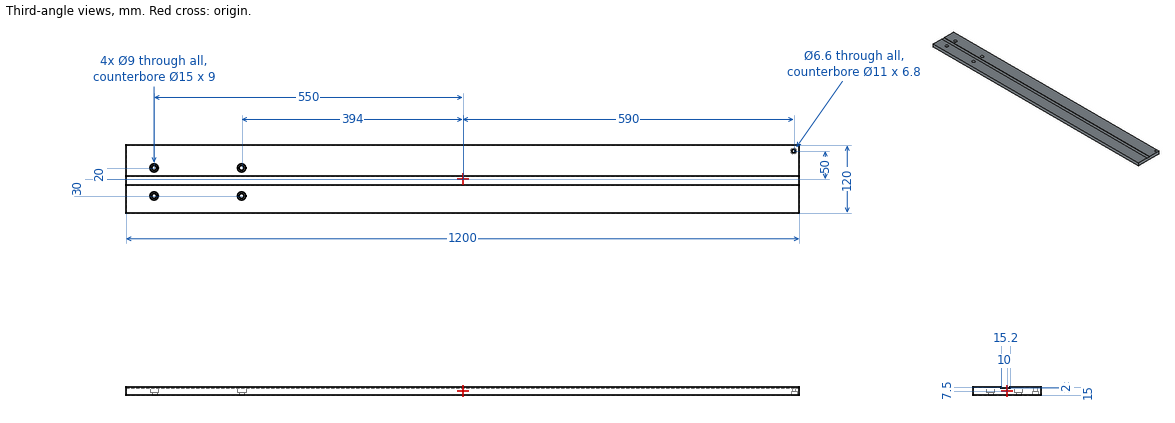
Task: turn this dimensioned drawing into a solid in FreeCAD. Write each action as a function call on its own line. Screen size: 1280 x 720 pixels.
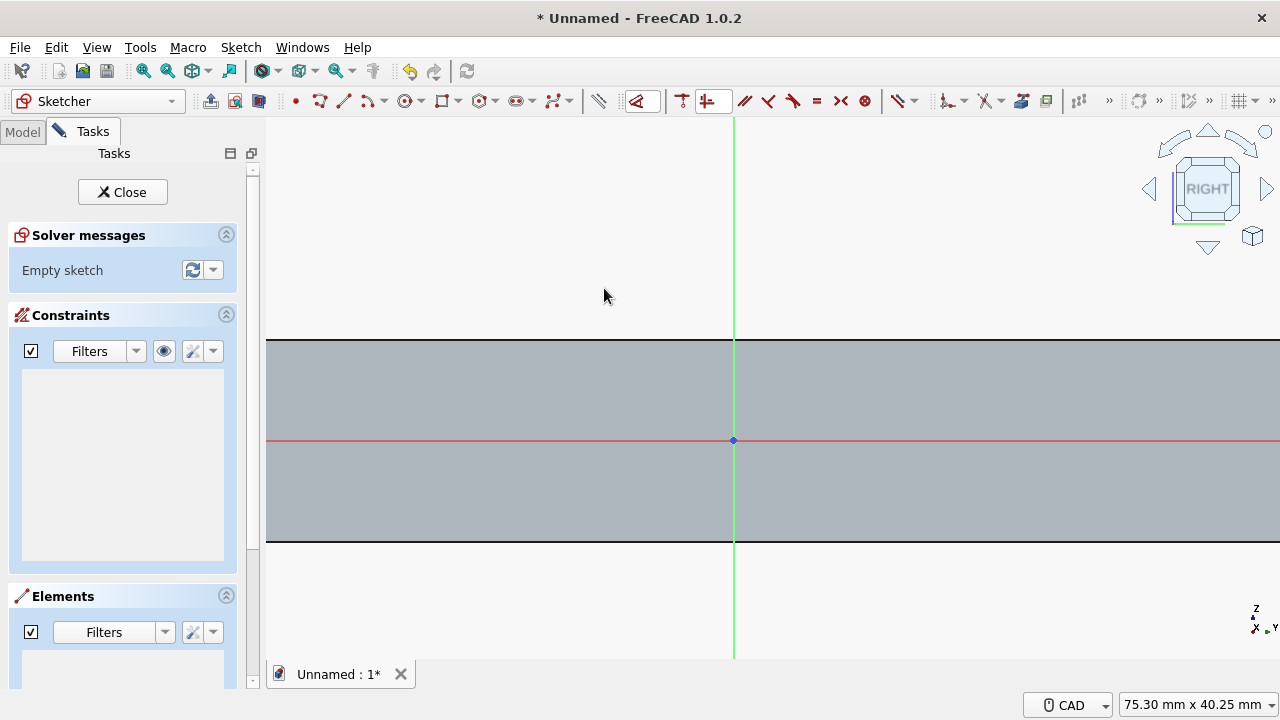
scroll(700, 392, up, 5)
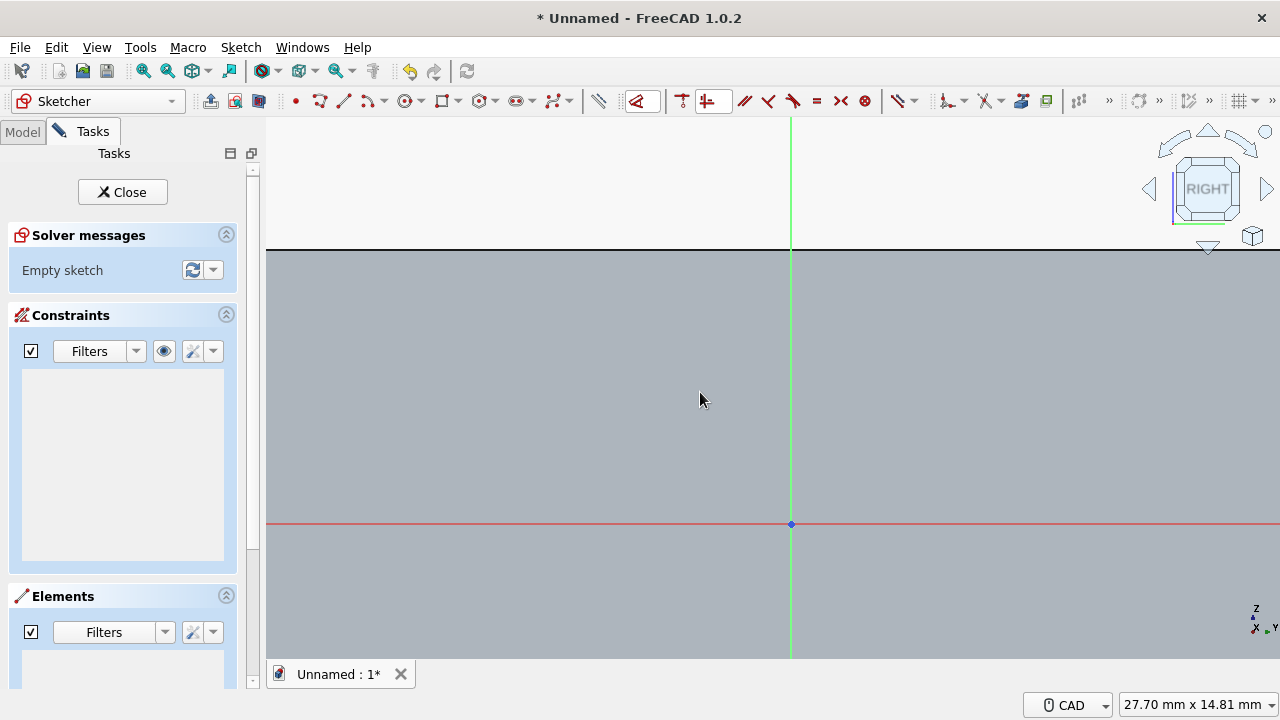
click(442, 102)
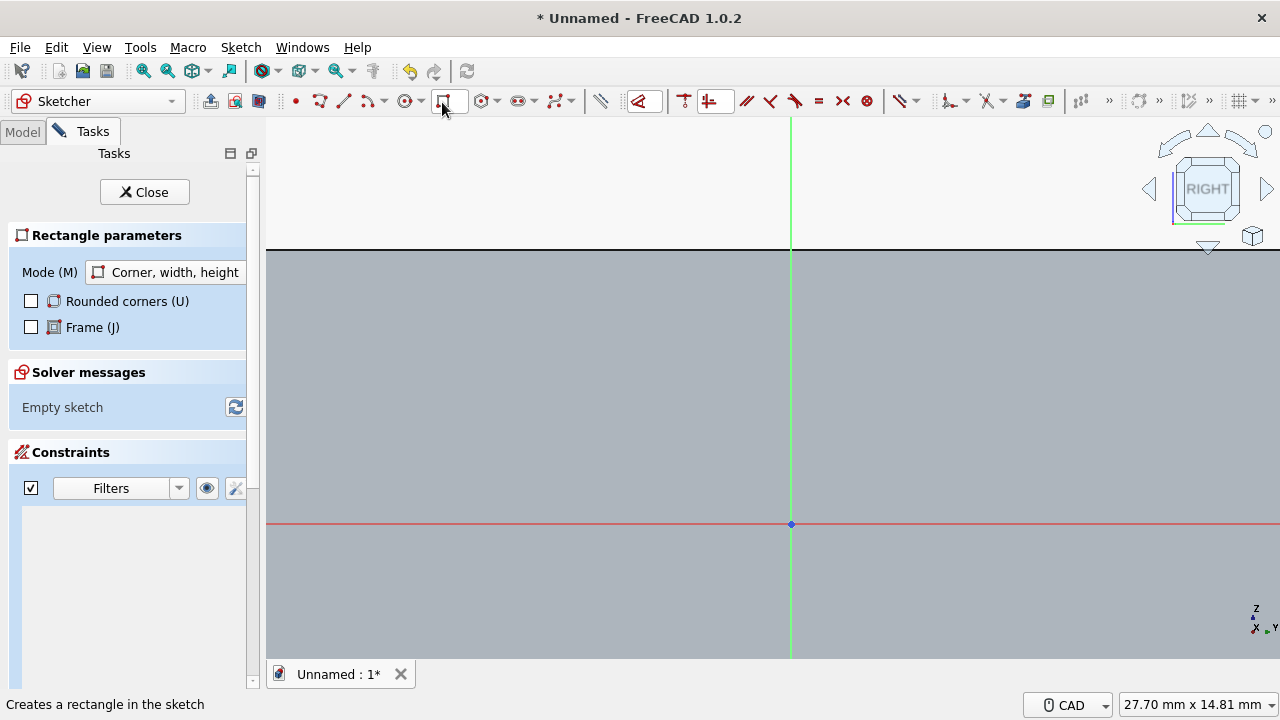
click(425, 250)
move(982, 323)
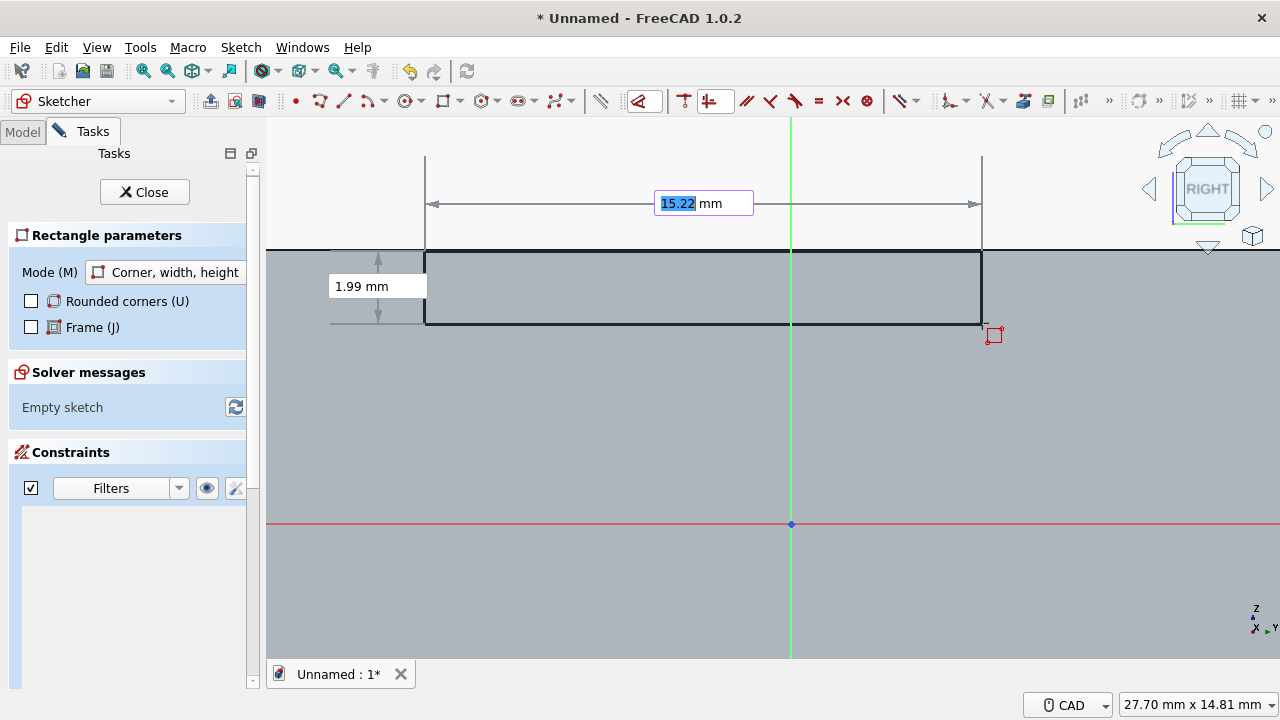
text(15.2)
key(Tab)
text(2)
key(Return)
key(Escape)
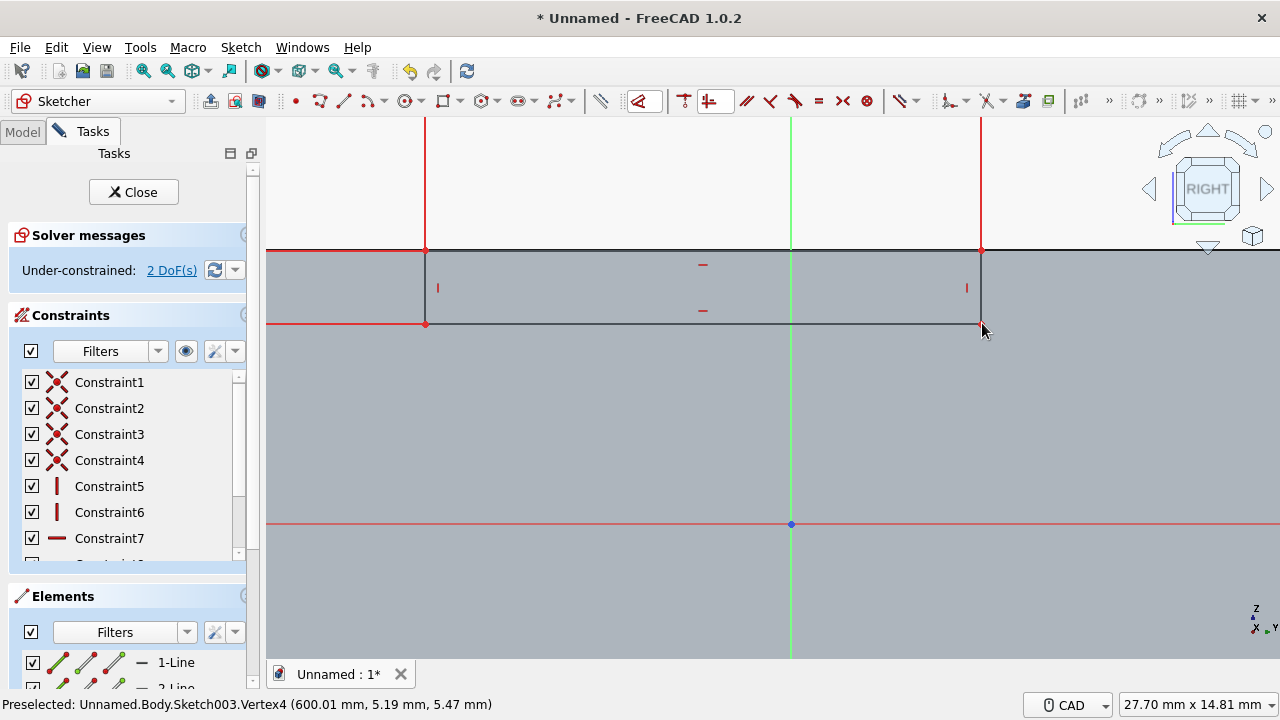
click(425, 251)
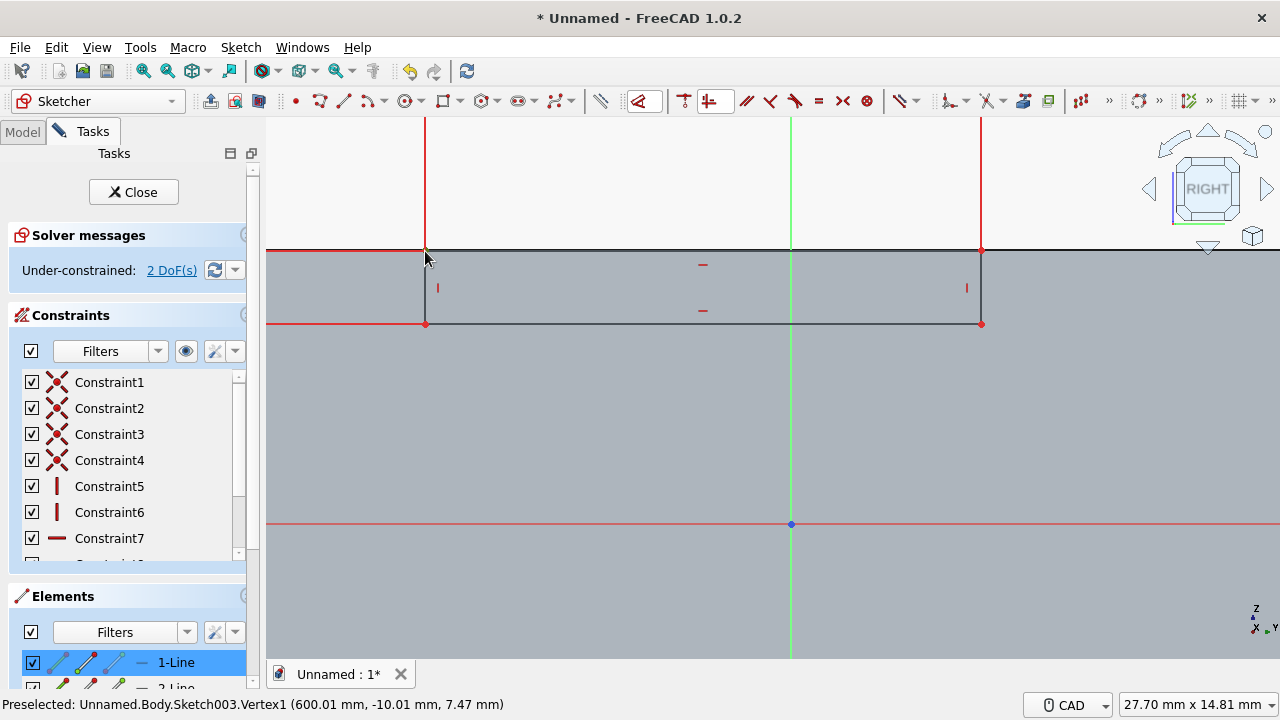
click(656, 102)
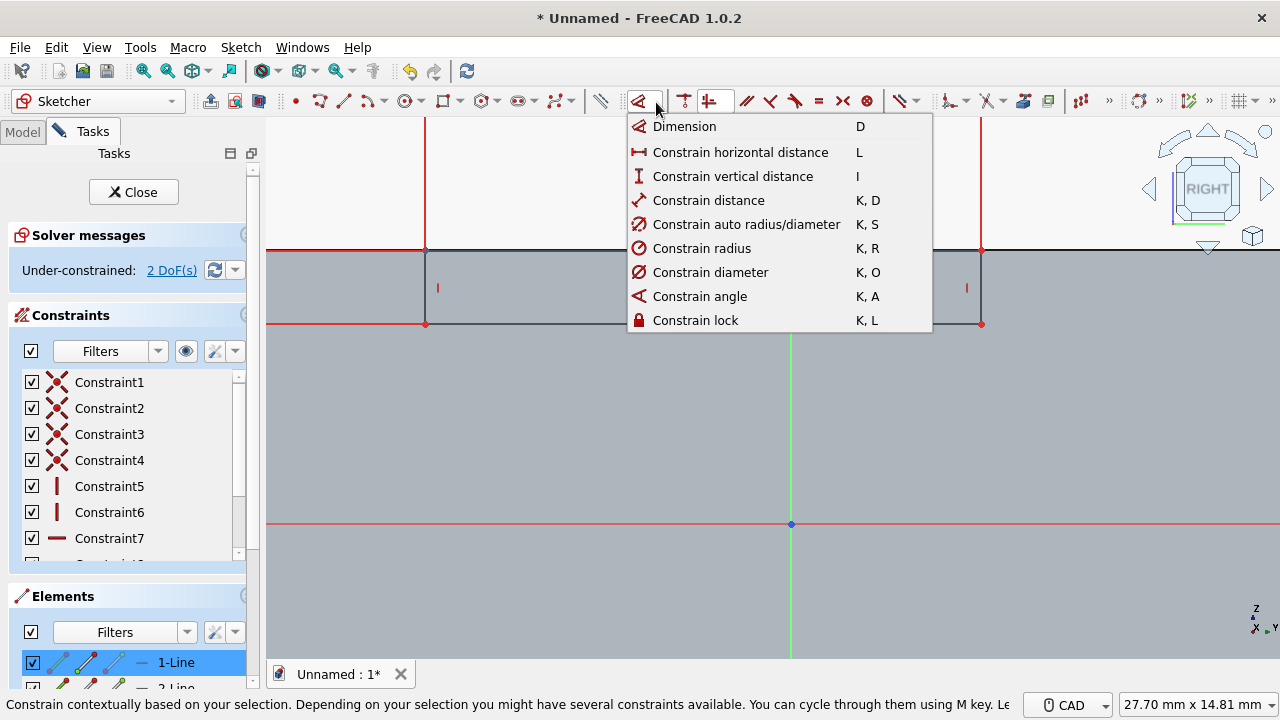
click(780, 152)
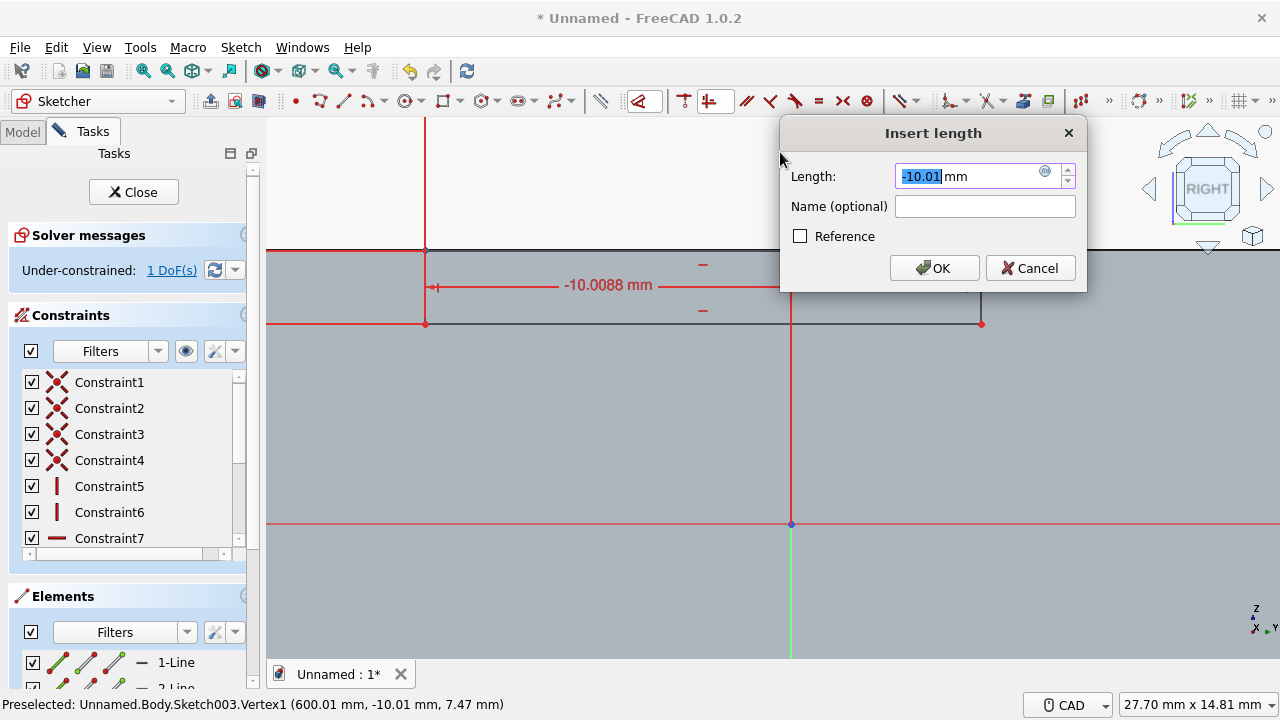
text(-10)
key(Return)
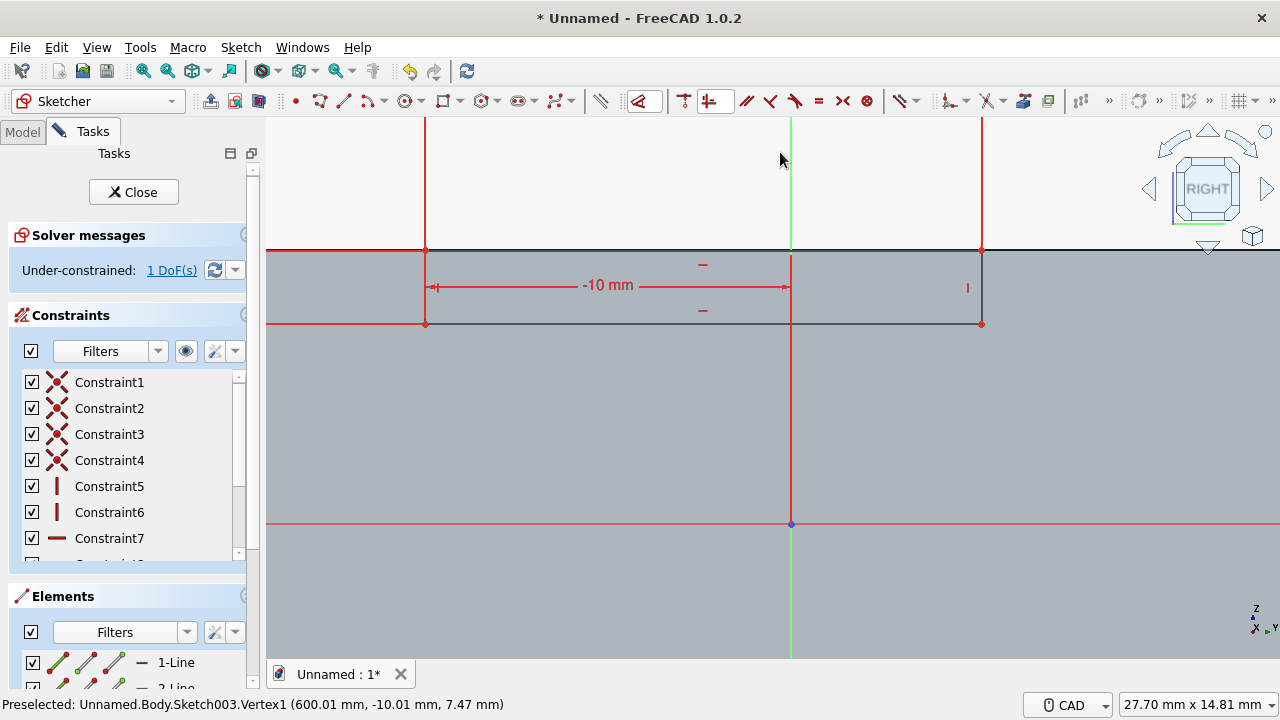
click(425, 251)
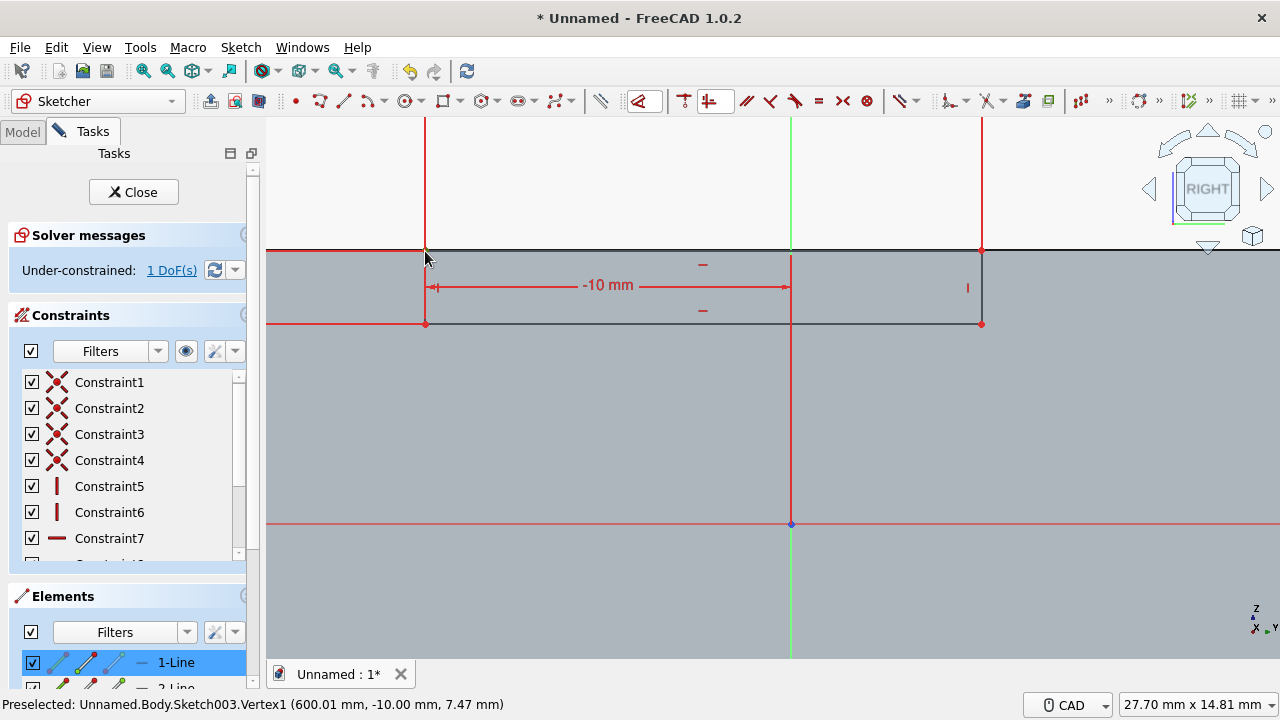
click(656, 102)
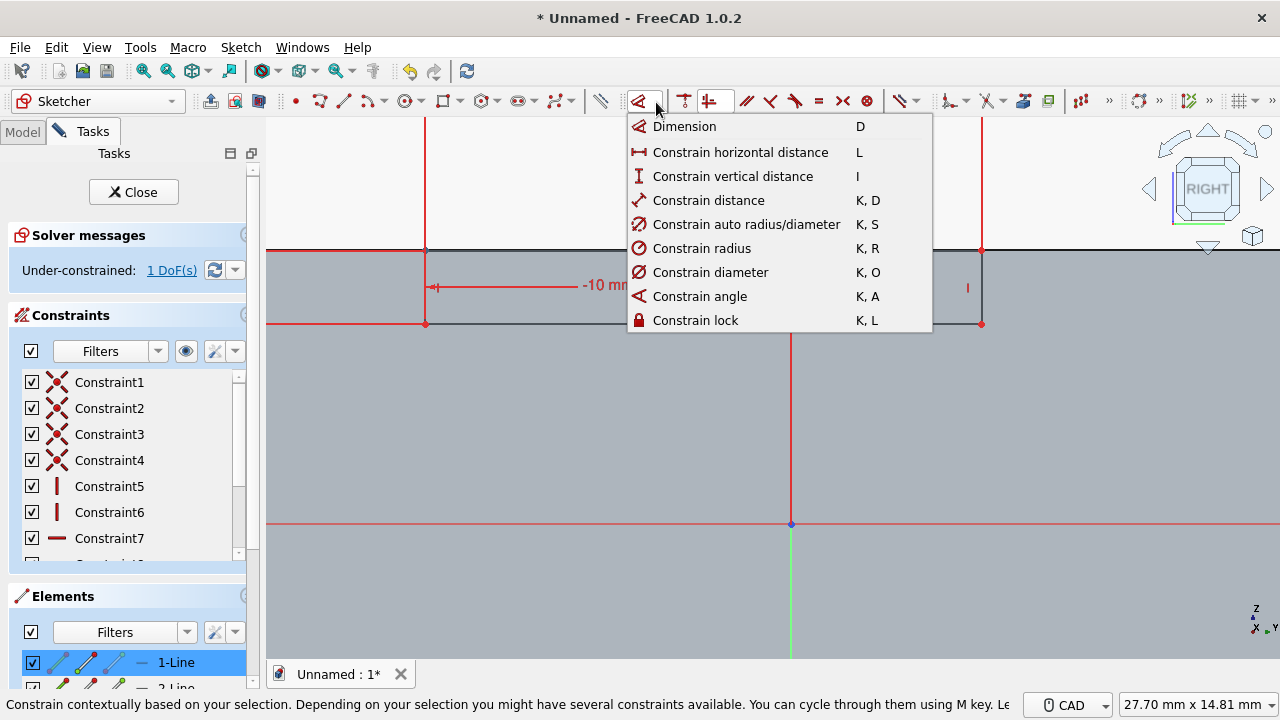
click(780, 176)